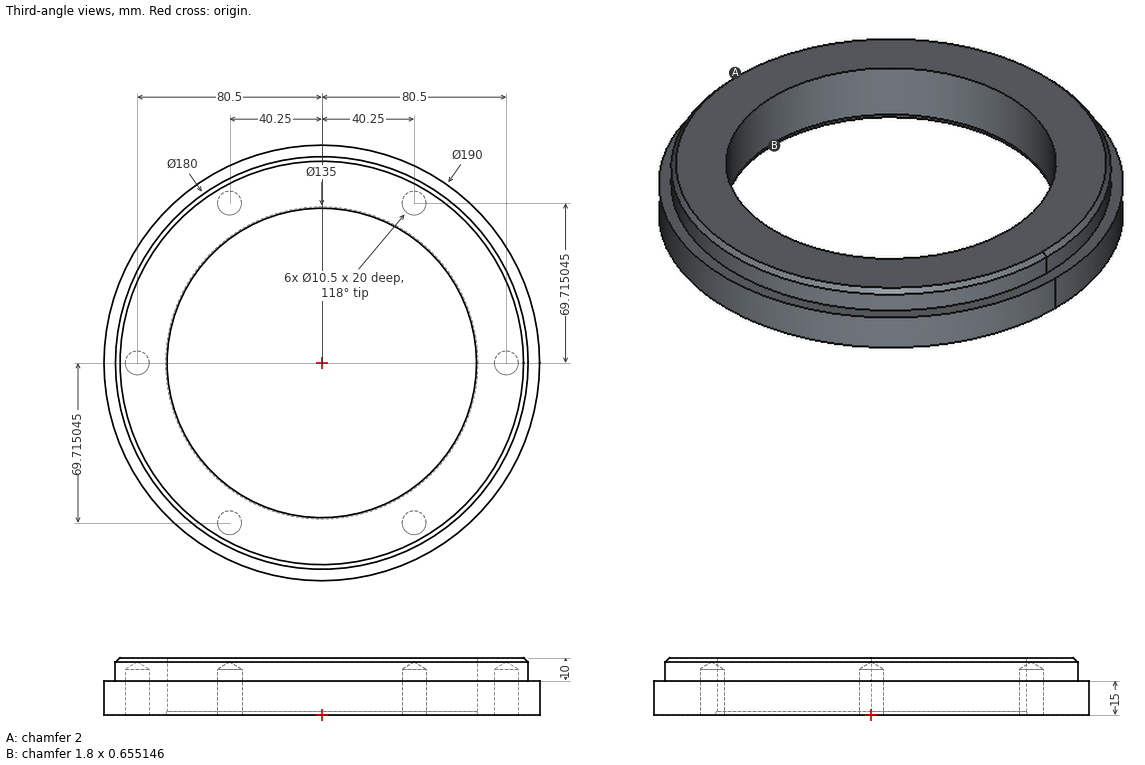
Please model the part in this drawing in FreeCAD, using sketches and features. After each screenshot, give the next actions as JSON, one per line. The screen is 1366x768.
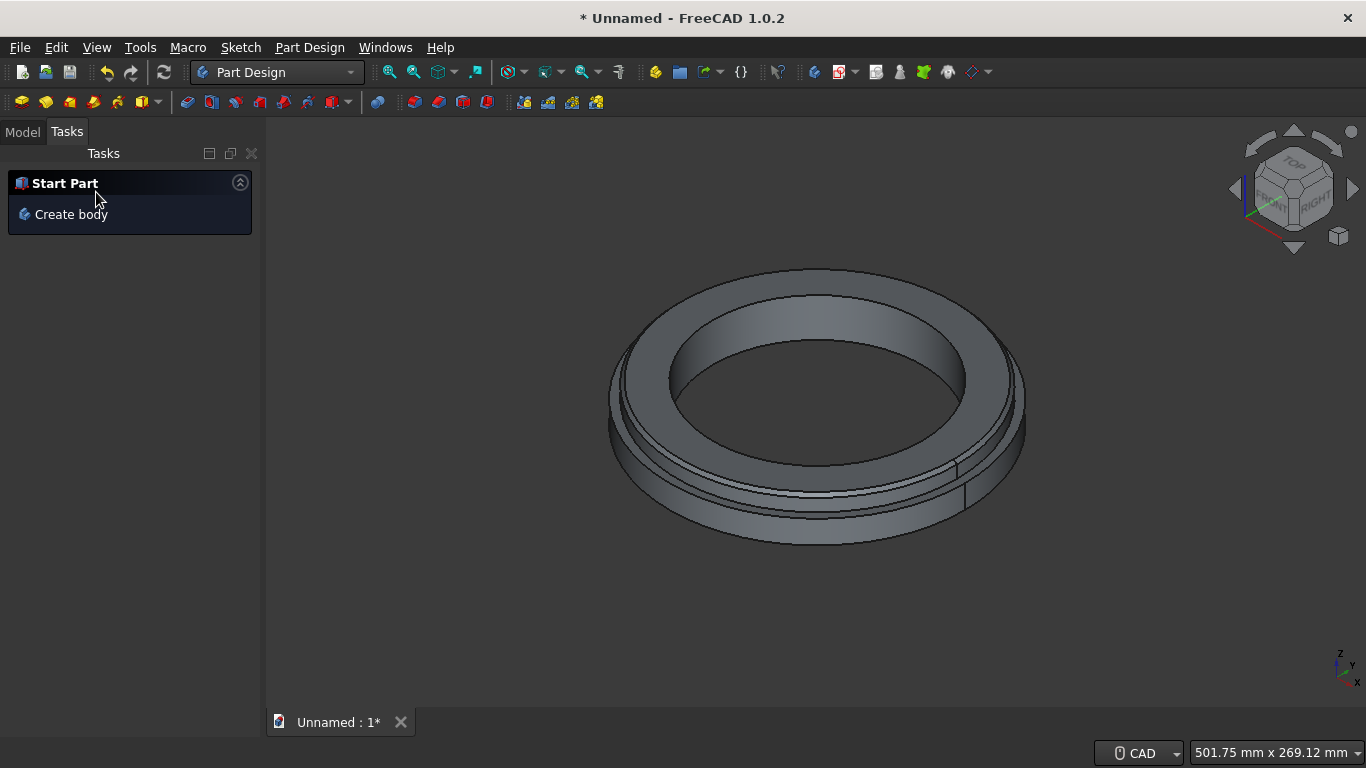
{"action": "key", "text": "2"}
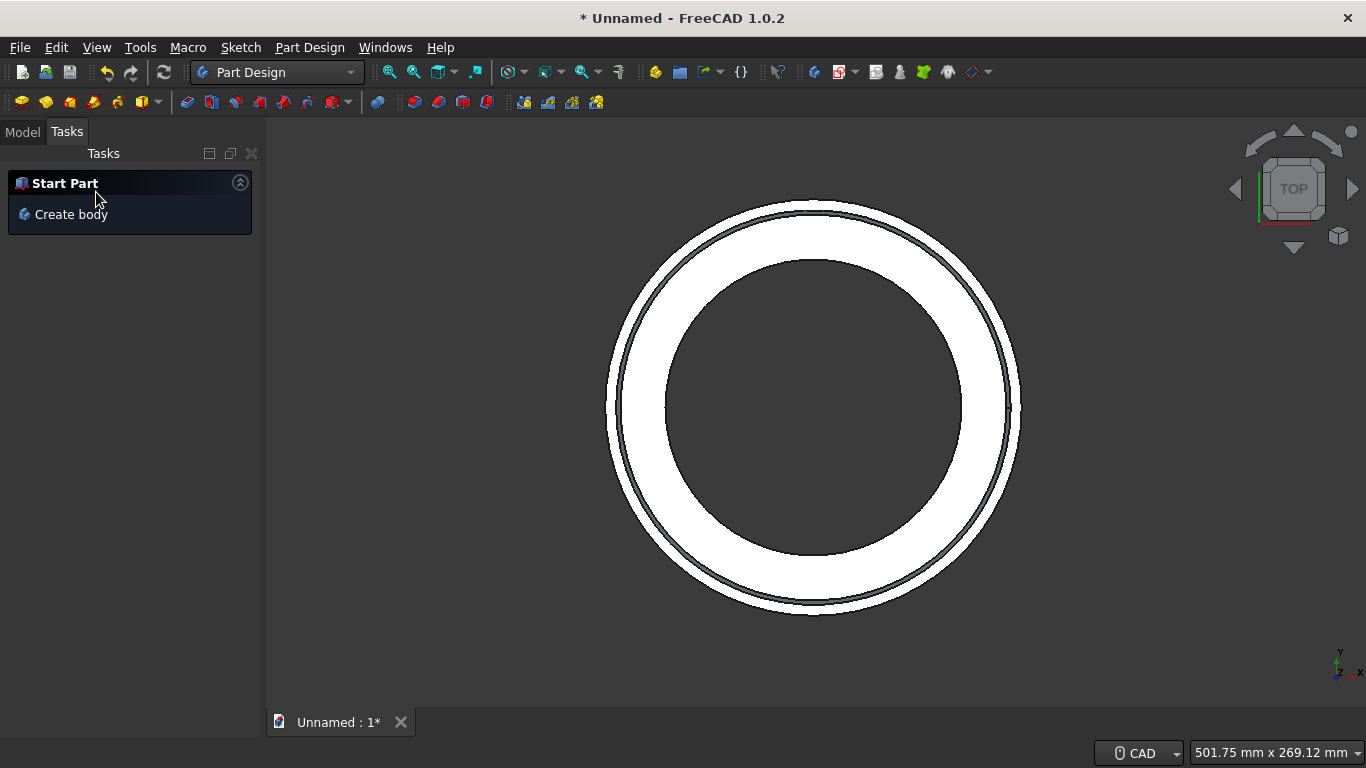
{"action": "key", "text": "1"}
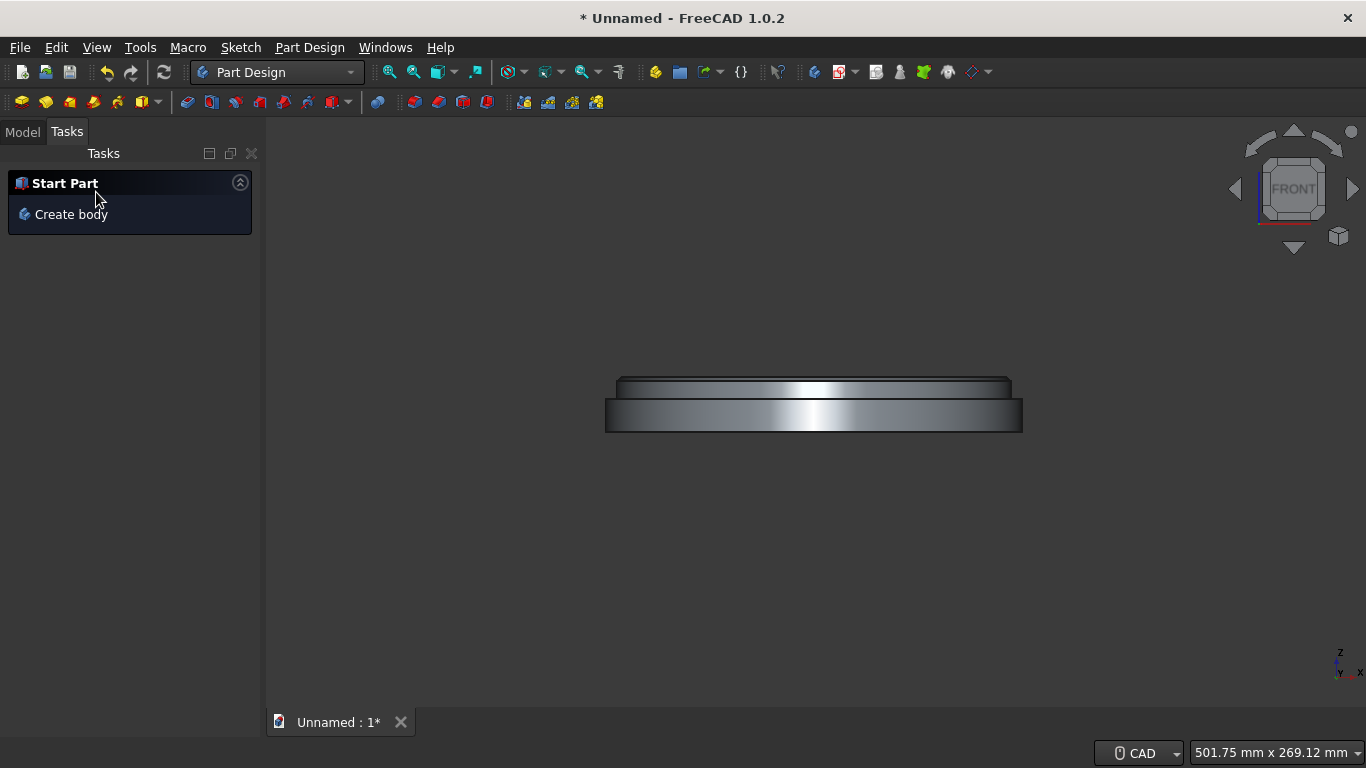
{"action": "left_click", "coordinate": [390, 72]}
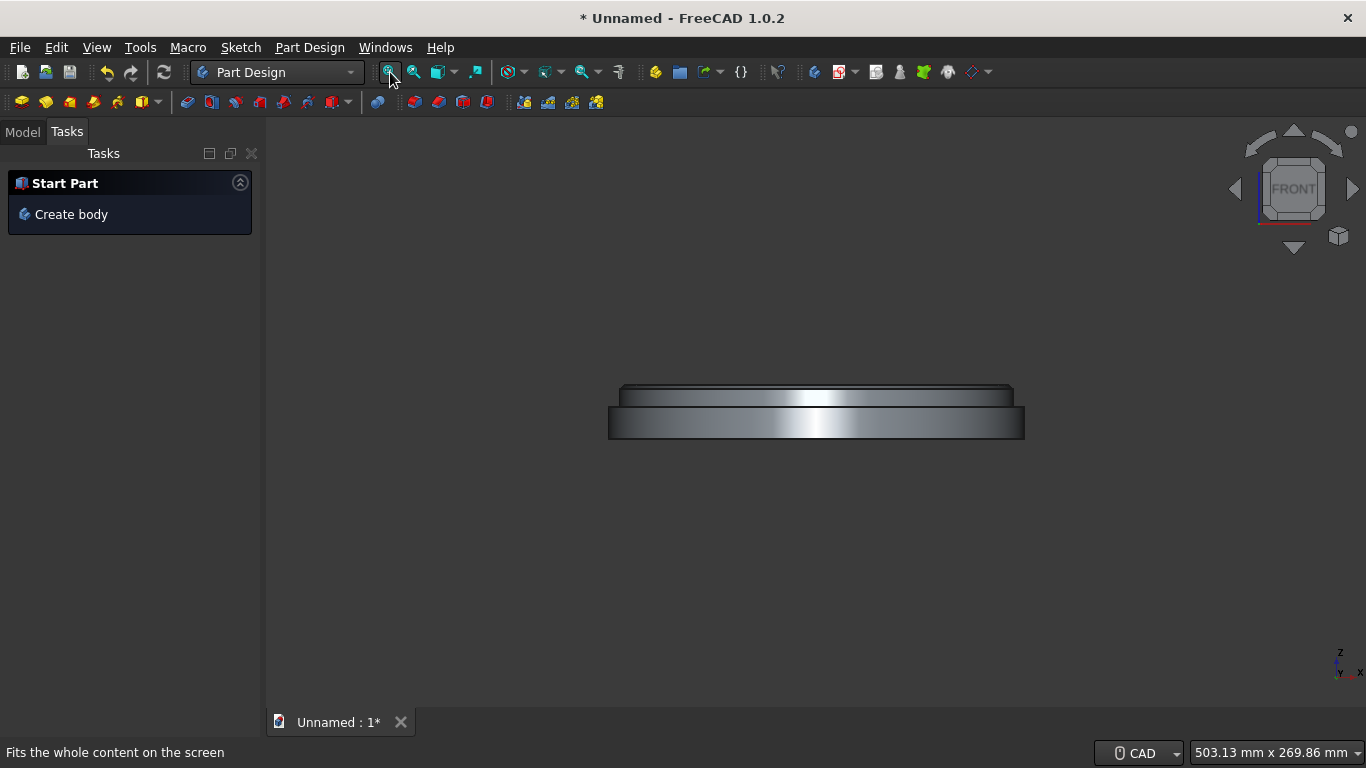
{"action": "key", "text": "3"}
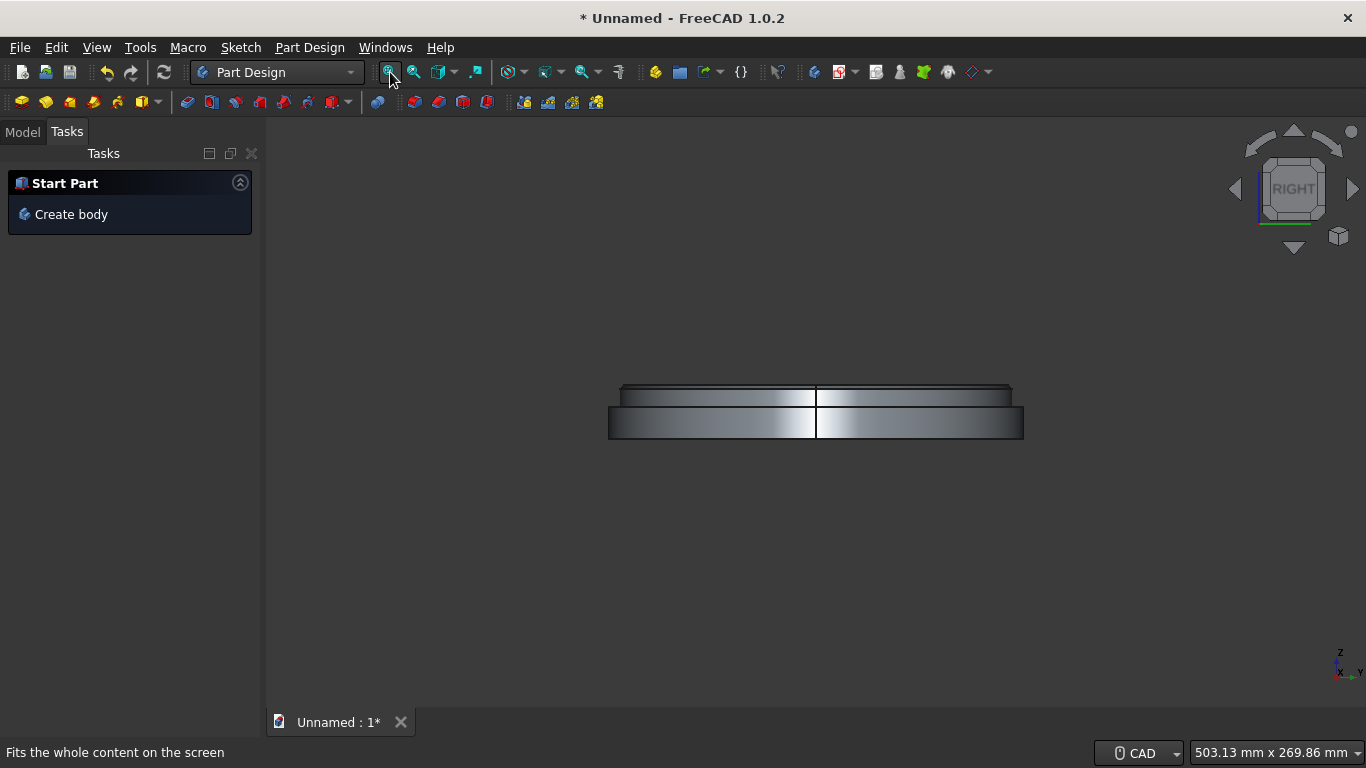
{"action": "left_click", "coordinate": [390, 72]}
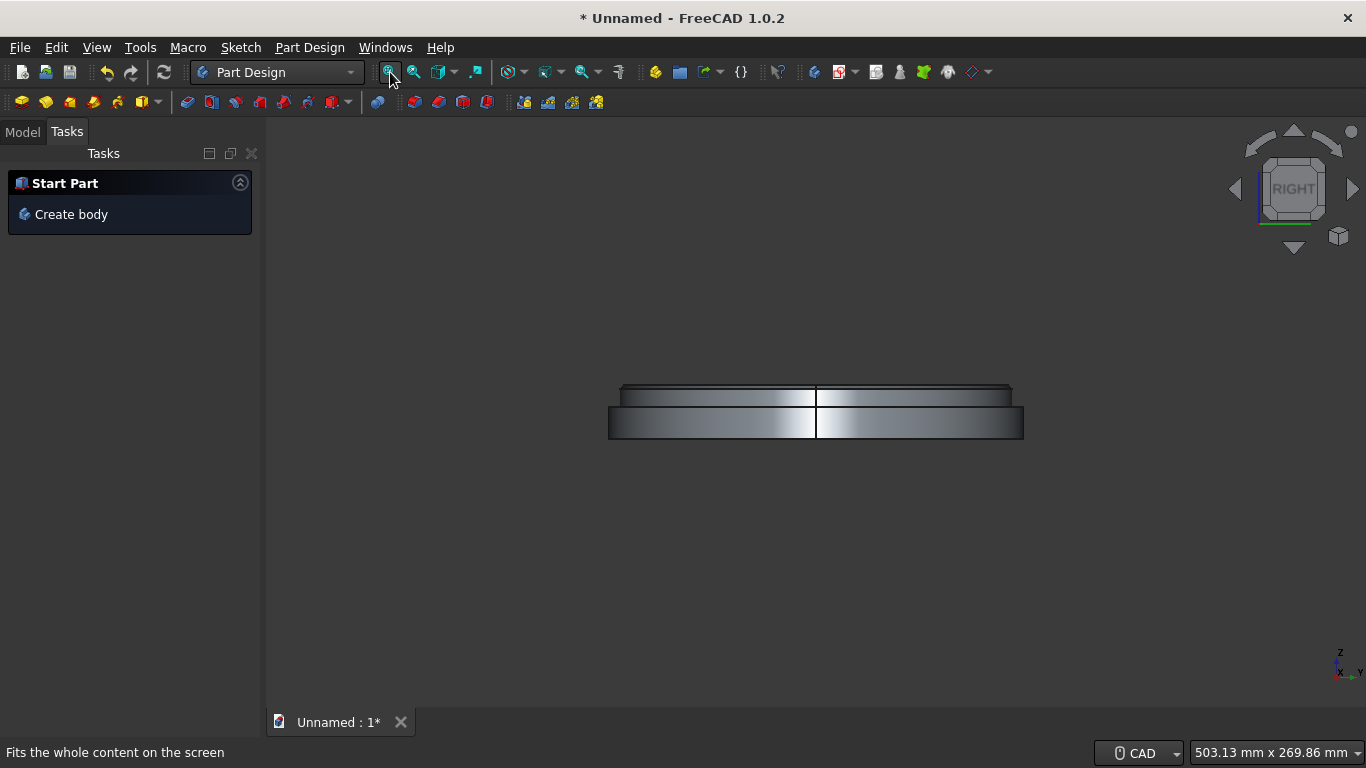
{"action": "key", "text": "5"}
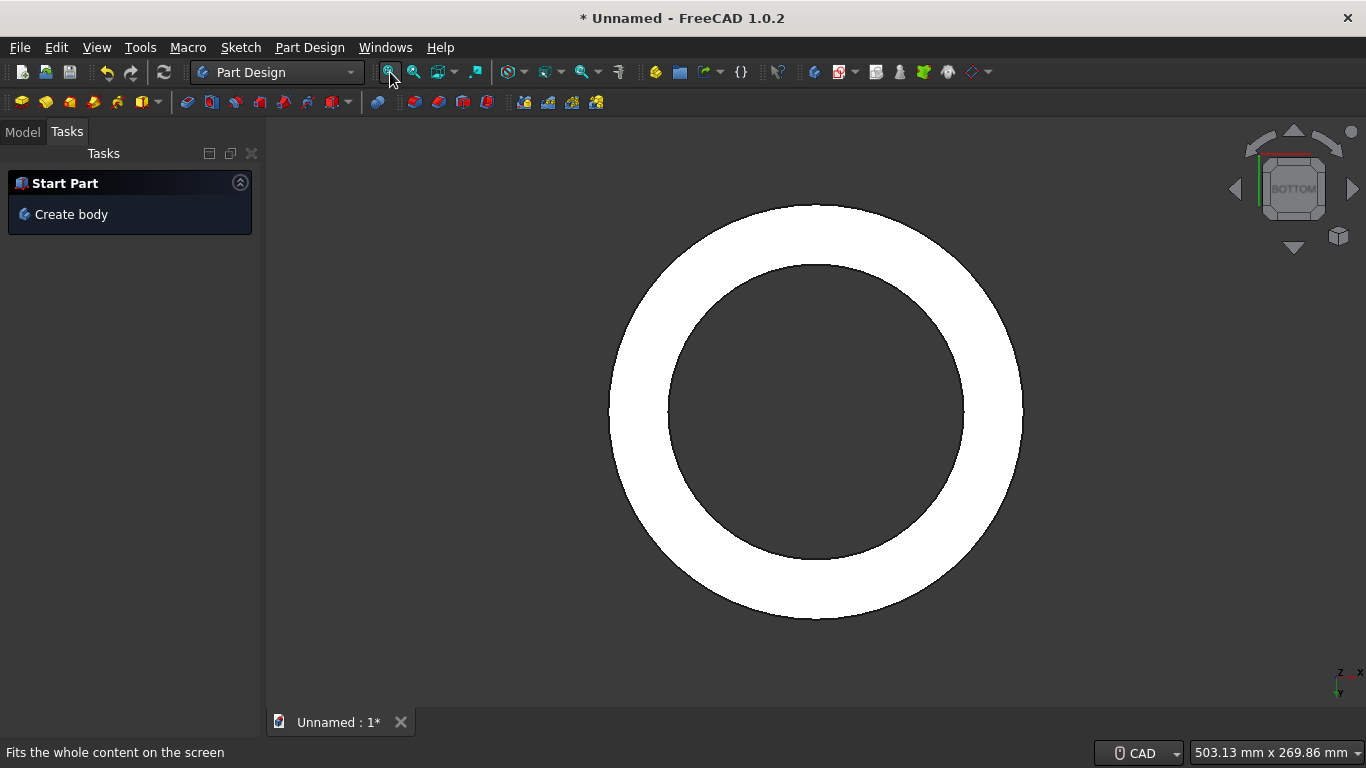
{"action": "left_click", "coordinate": [697, 498]}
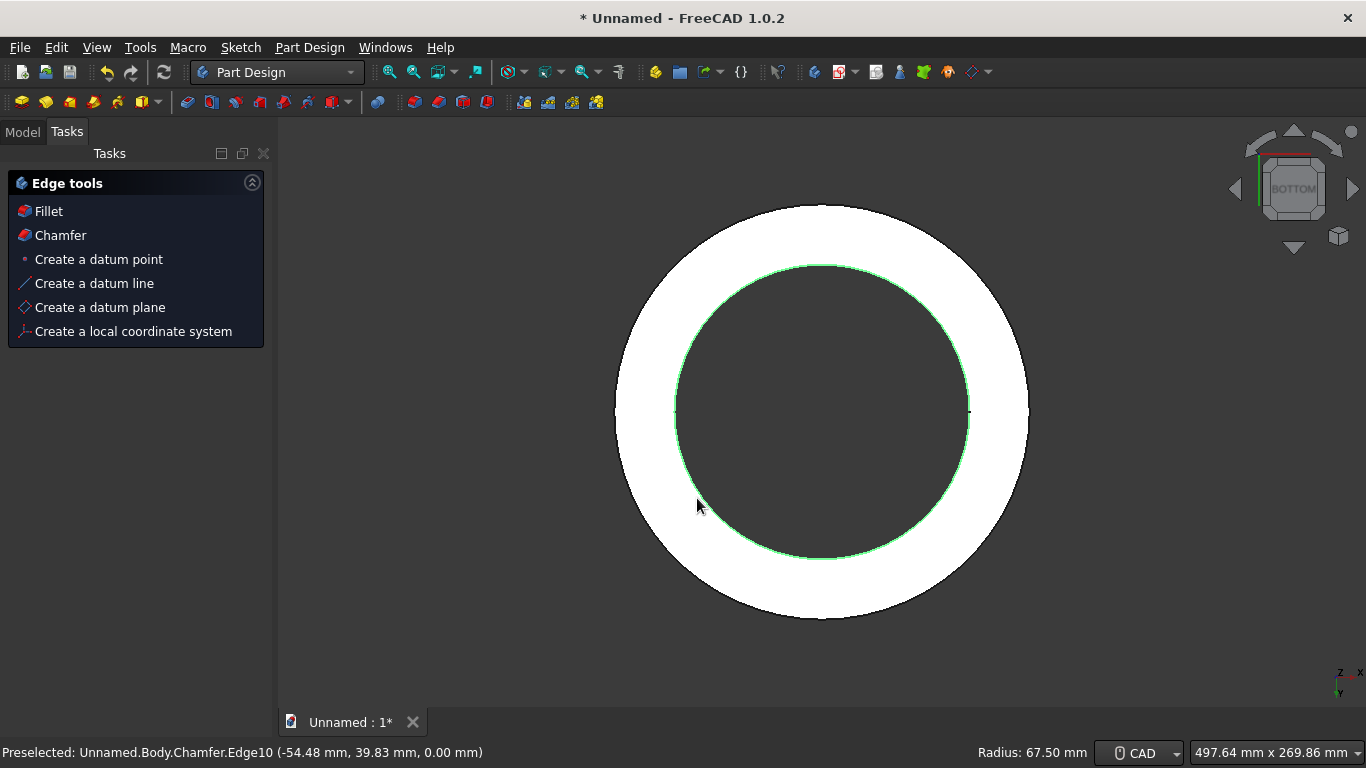
{"action": "left_click", "coordinate": [440, 102]}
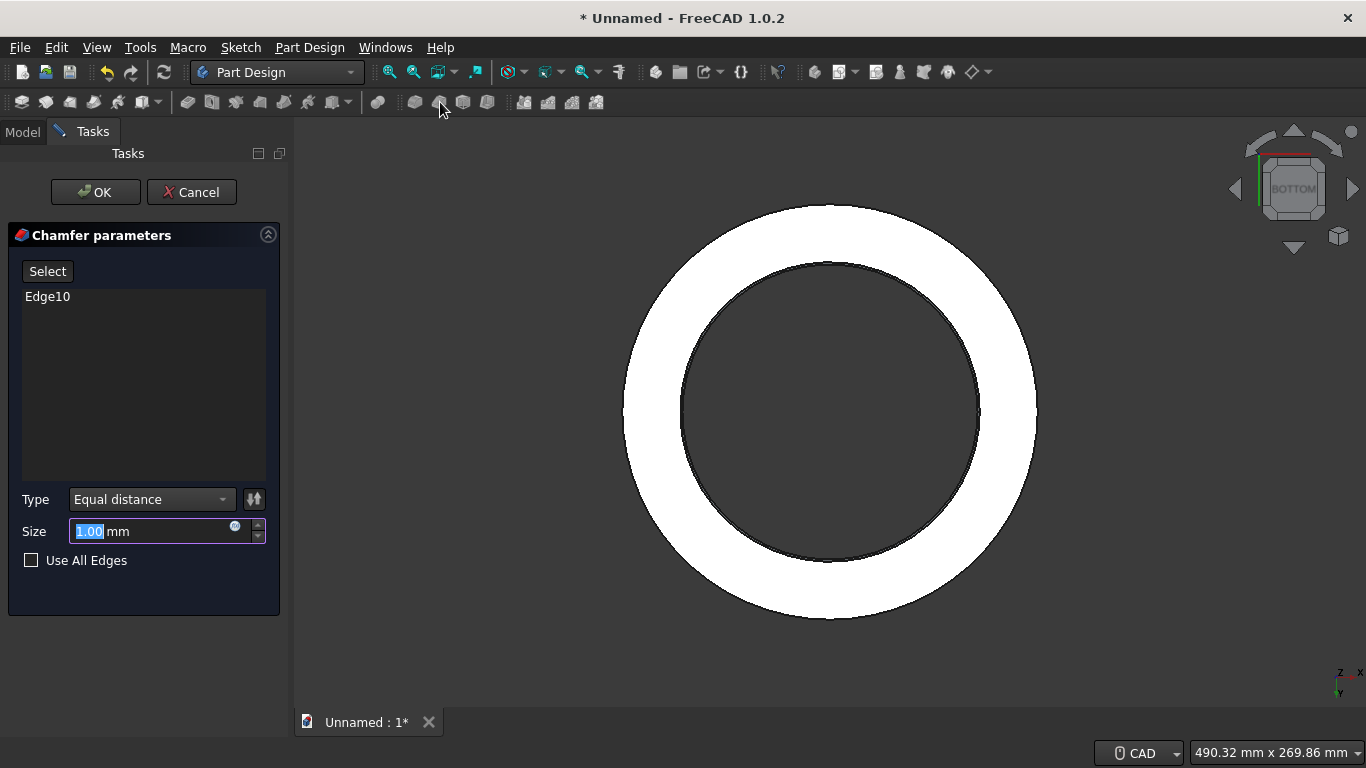
{"action": "type", "text": "1.8"}
{"action": "key", "text": "Tab"}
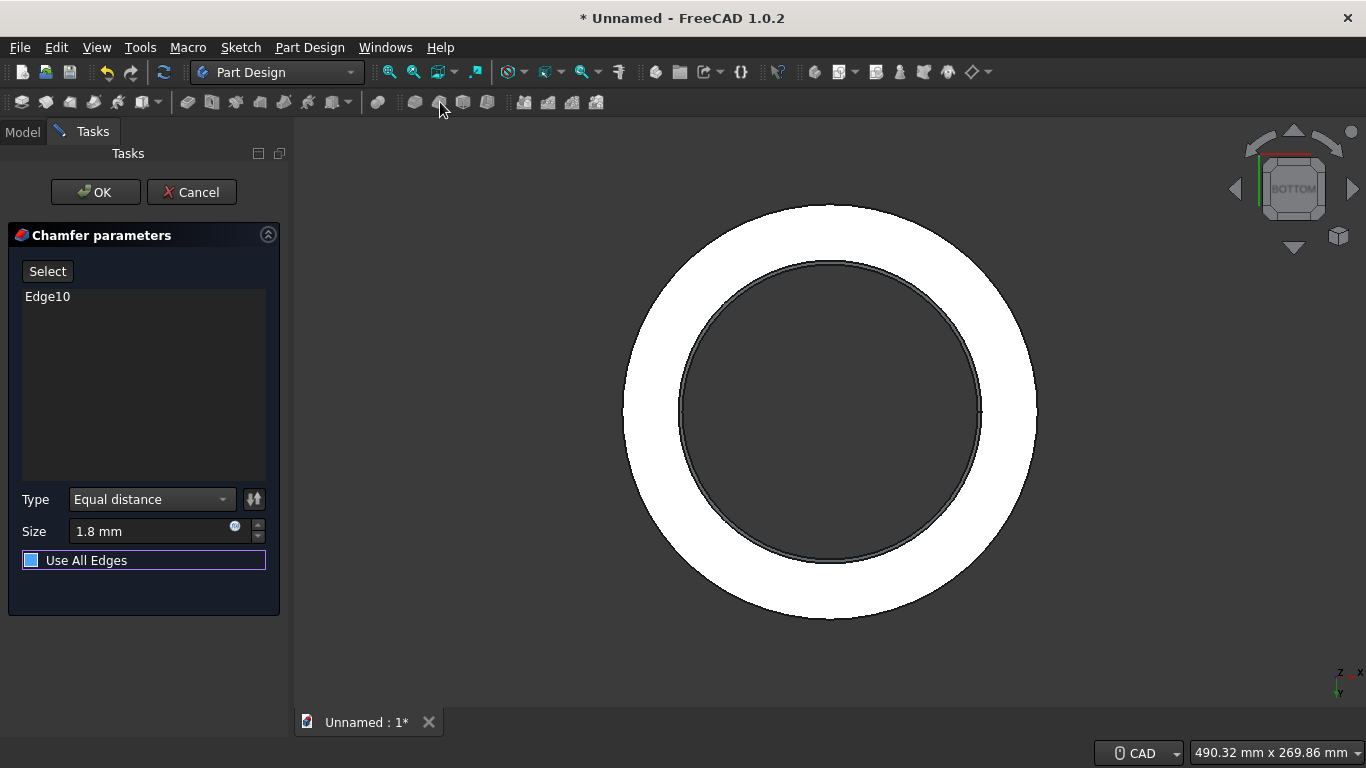
{"action": "left_click", "coordinate": [153, 500]}